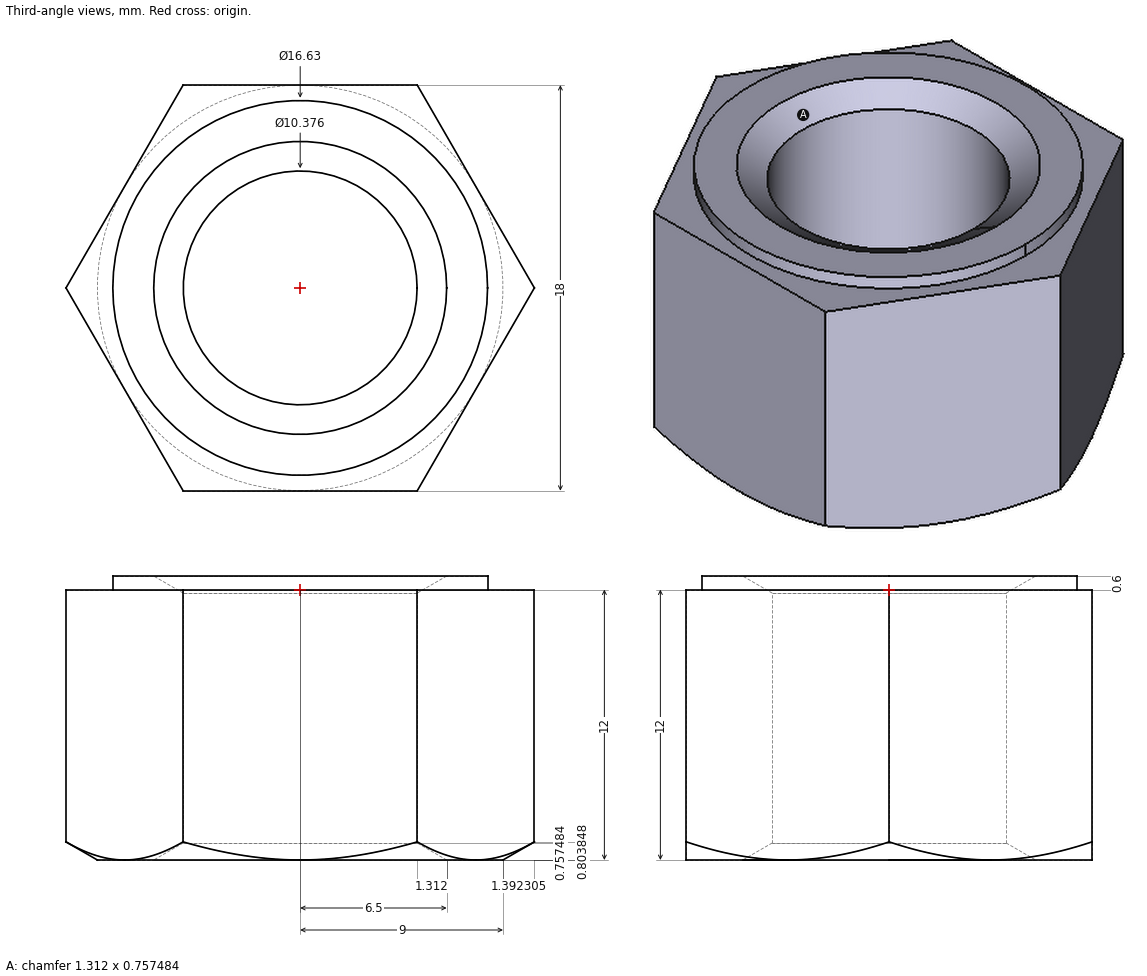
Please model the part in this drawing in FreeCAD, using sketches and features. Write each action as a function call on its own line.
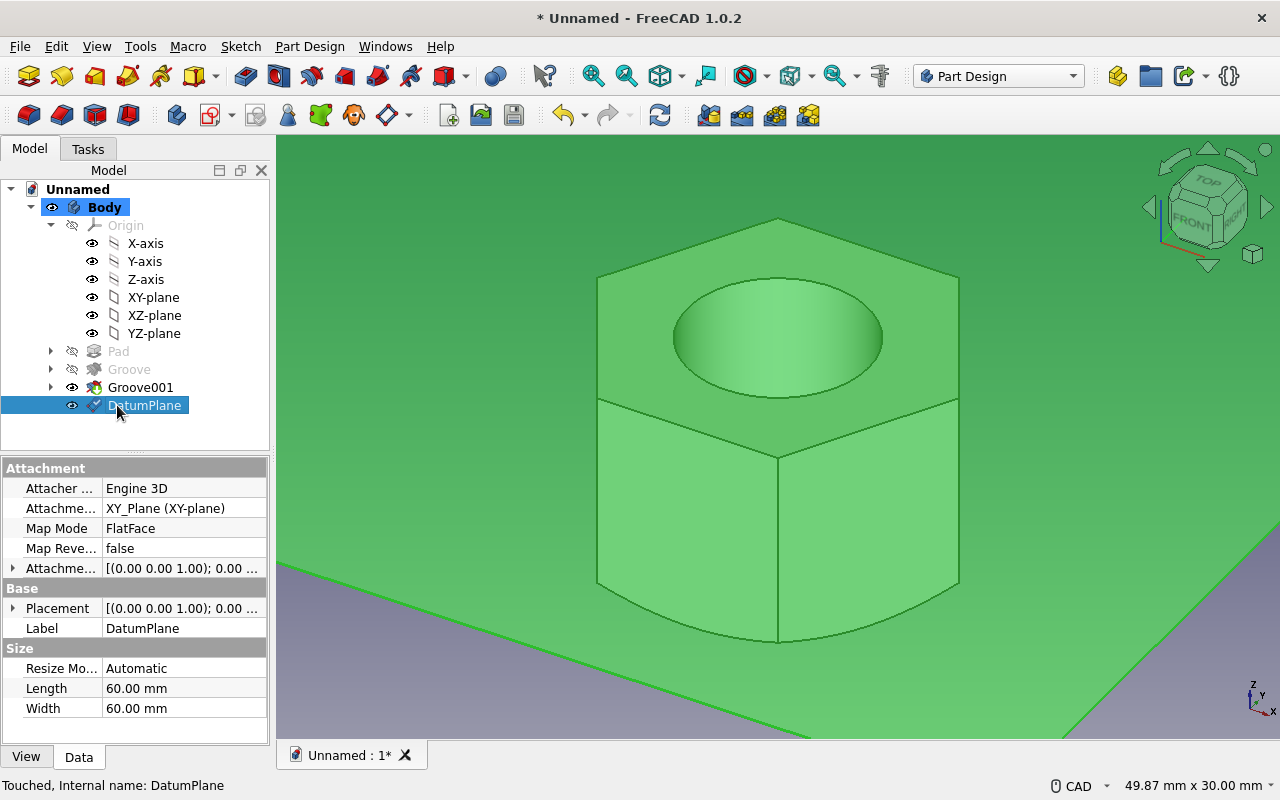
click(210, 116)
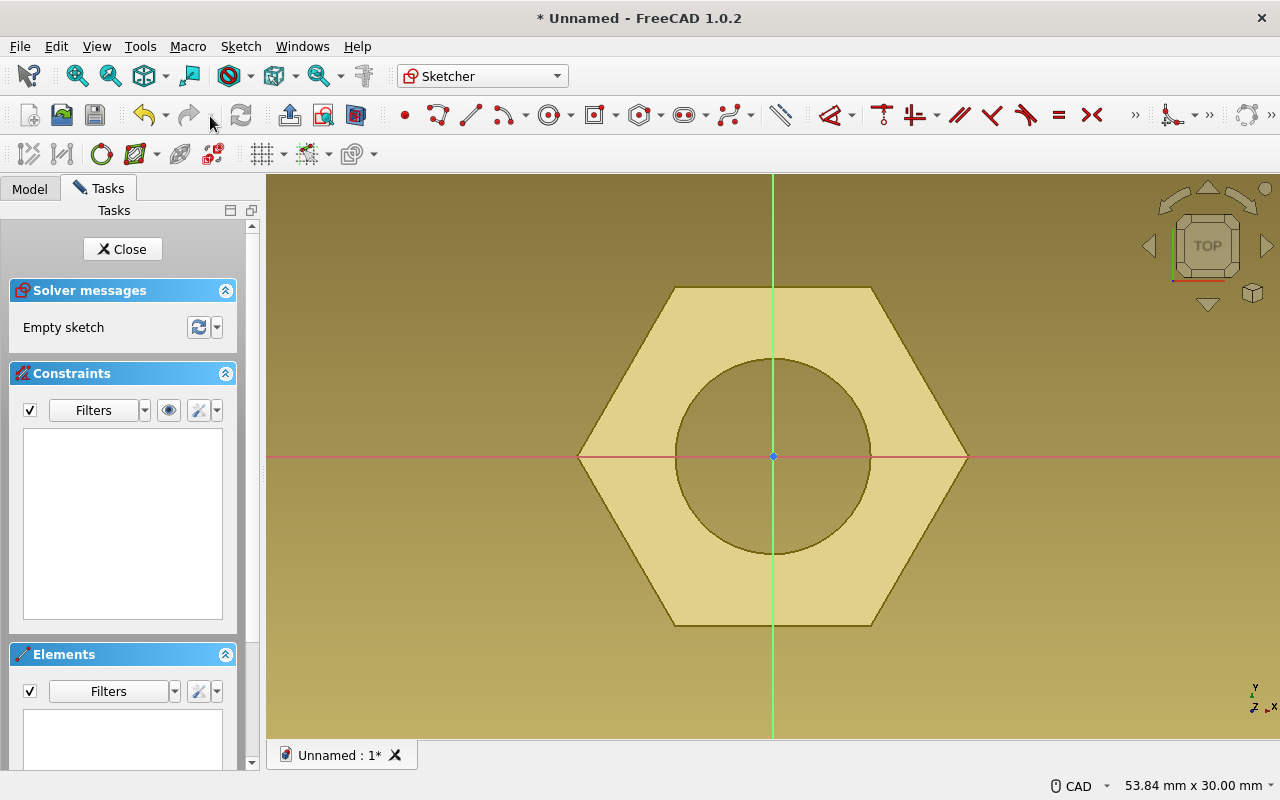
key(g)
key(c)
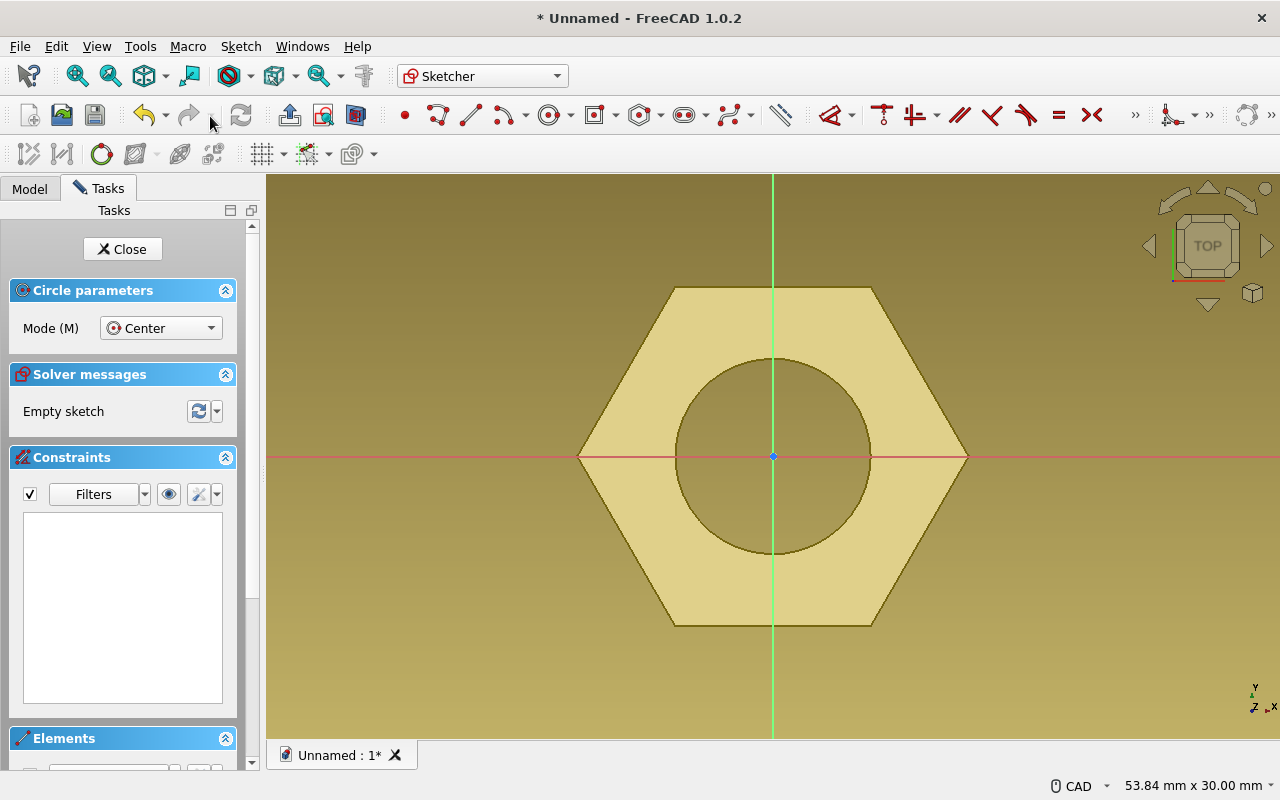
click(773, 456)
click(884, 346)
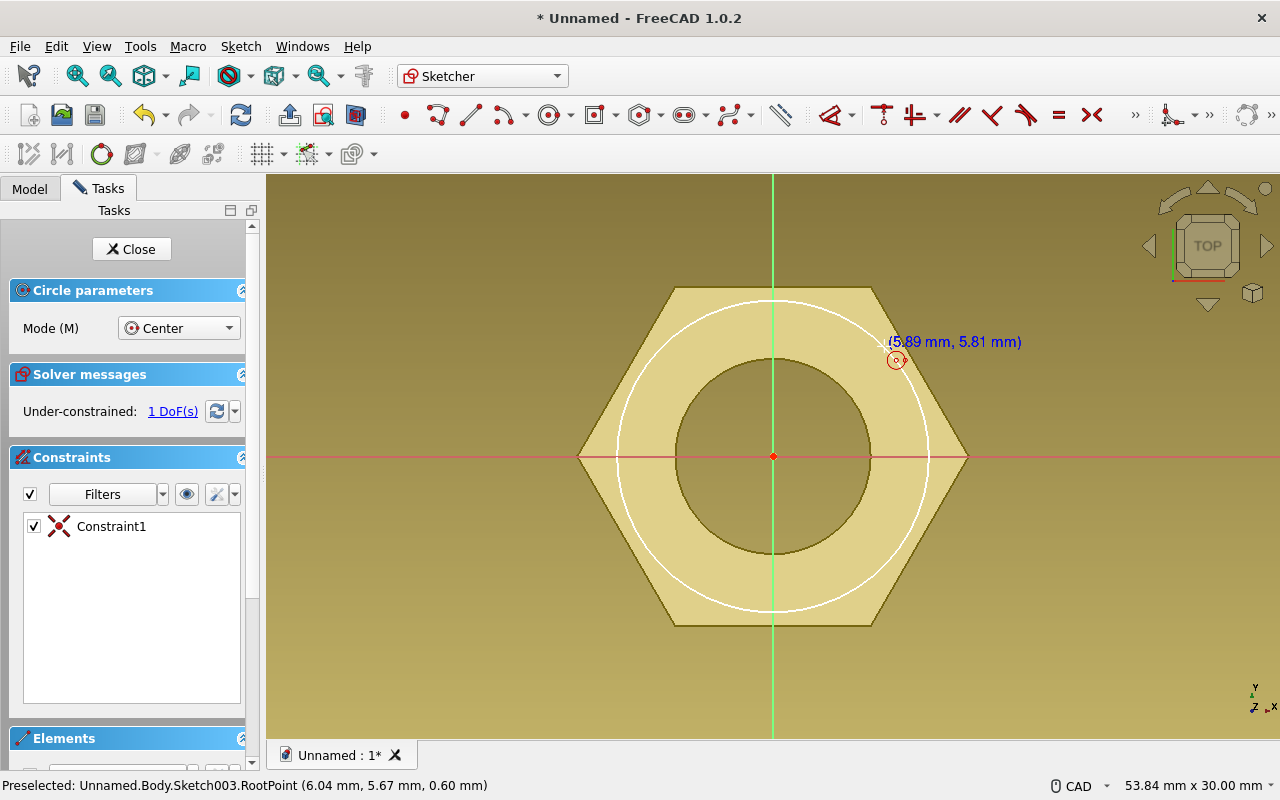
click(773, 456)
click(842, 387)
key(Escape)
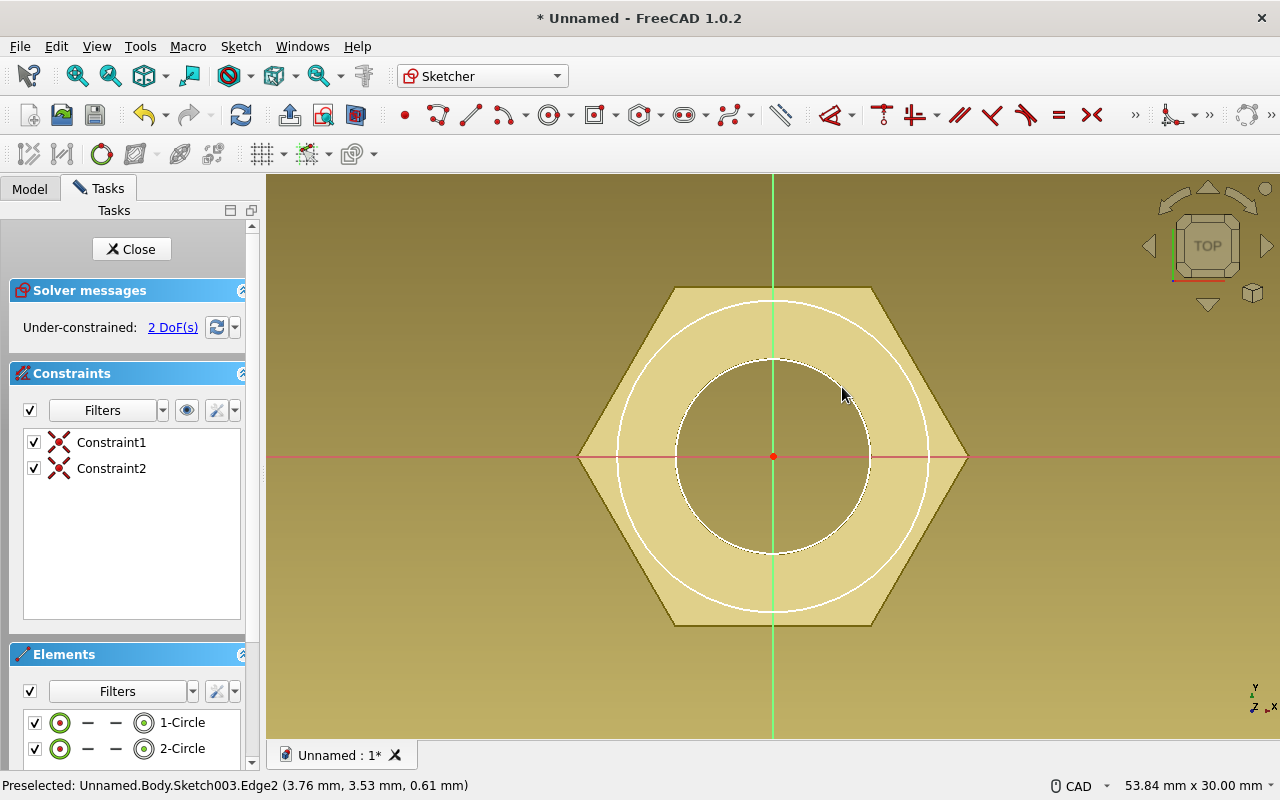
key(d)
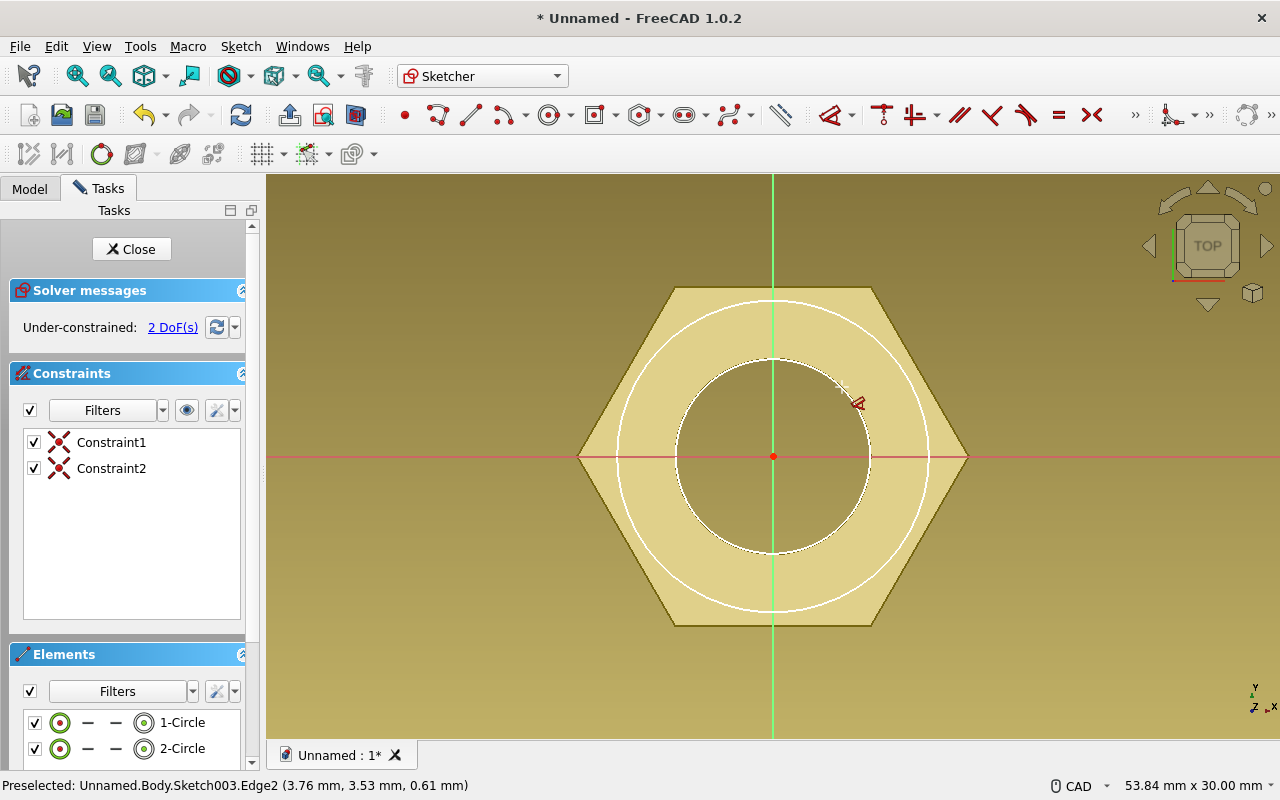
click(883, 346)
click(906, 323)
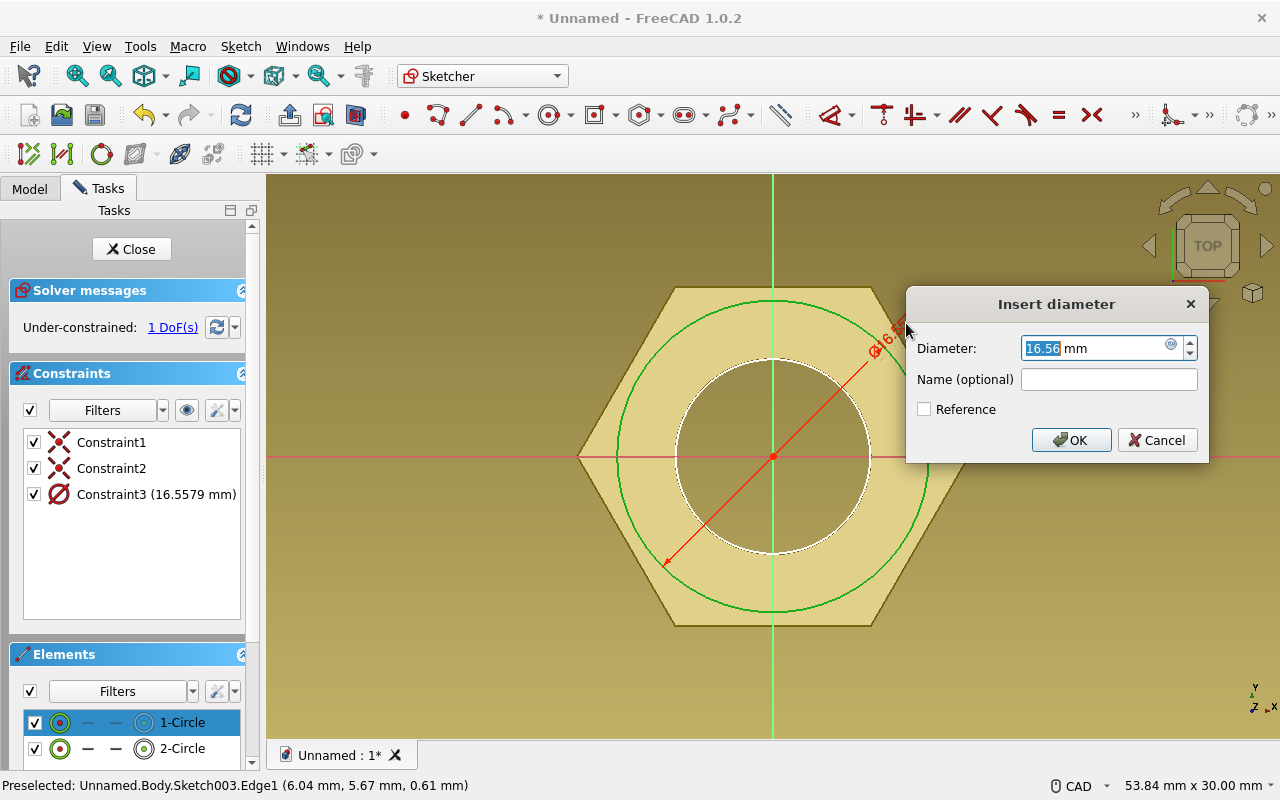
text(16.63)
key(Return)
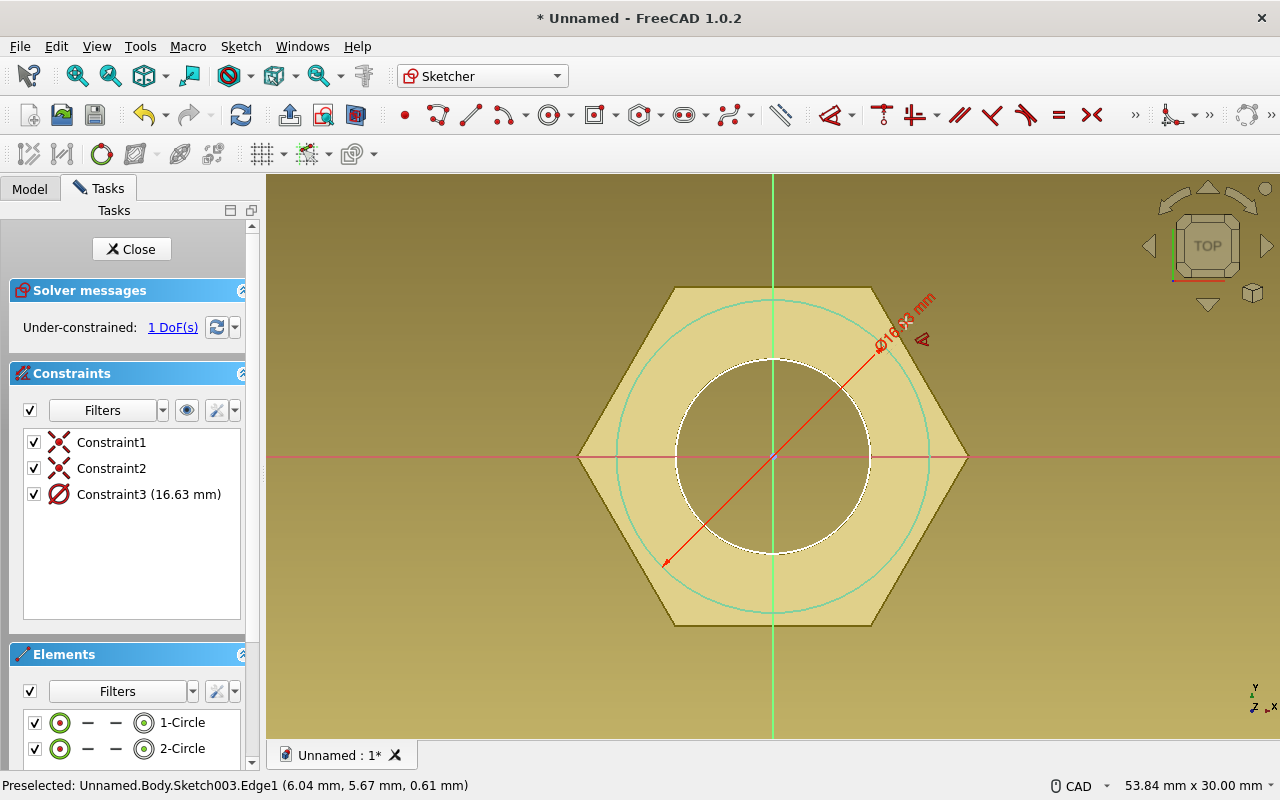
click(842, 388)
click(865, 365)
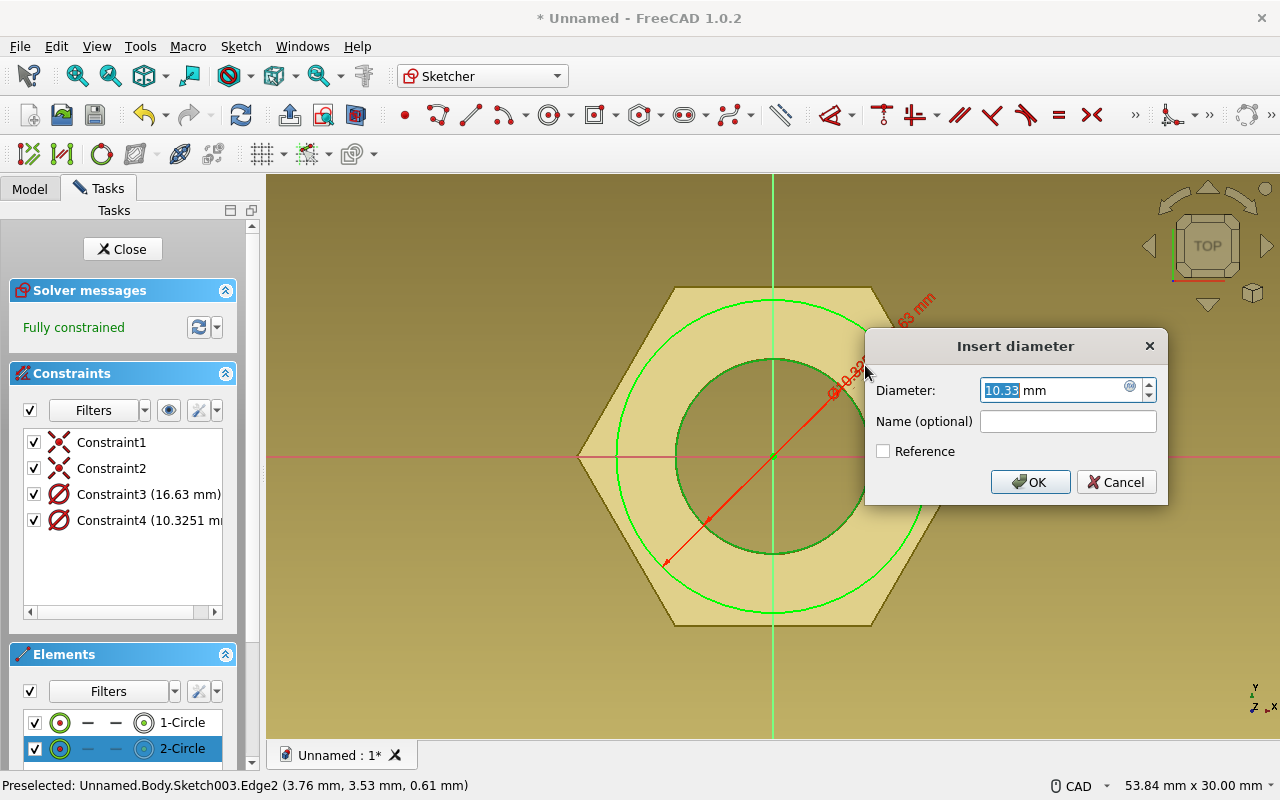
text(10.376)
key(Return)
key(Escape)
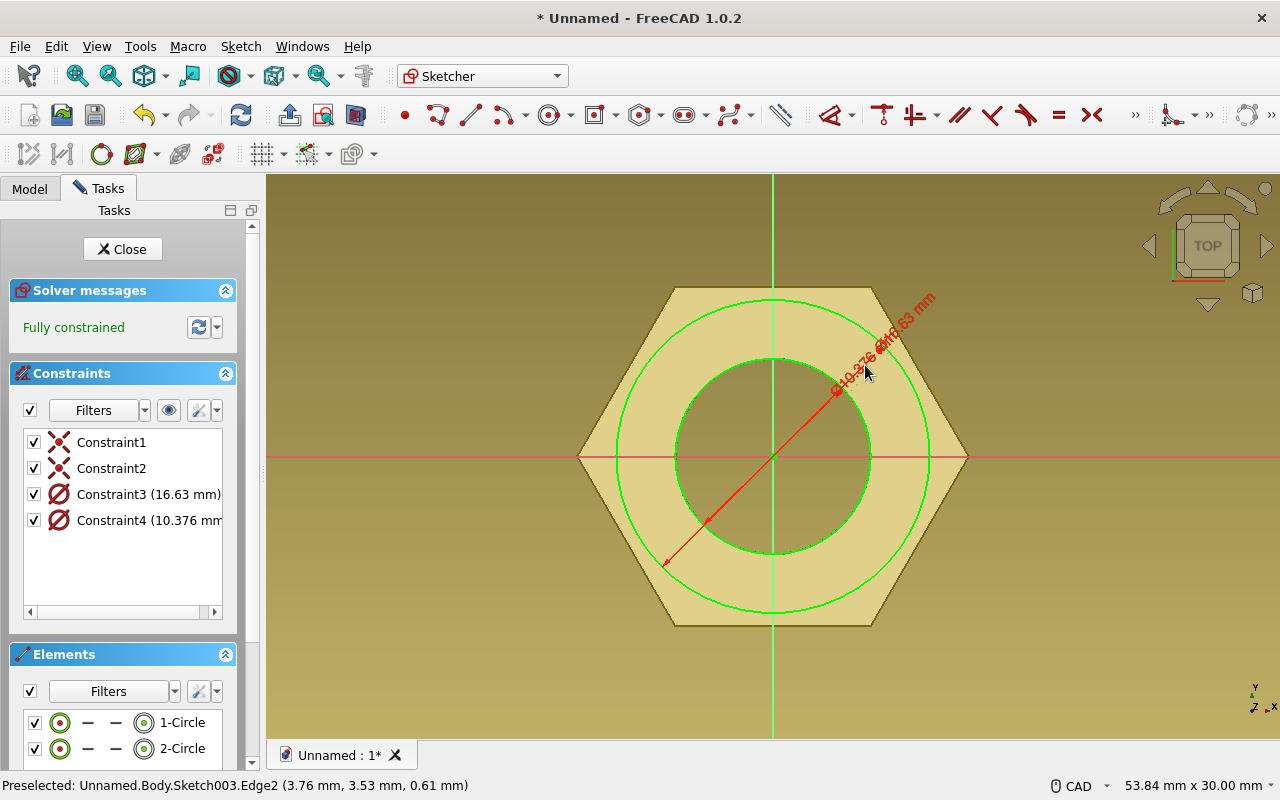
click(123, 249)